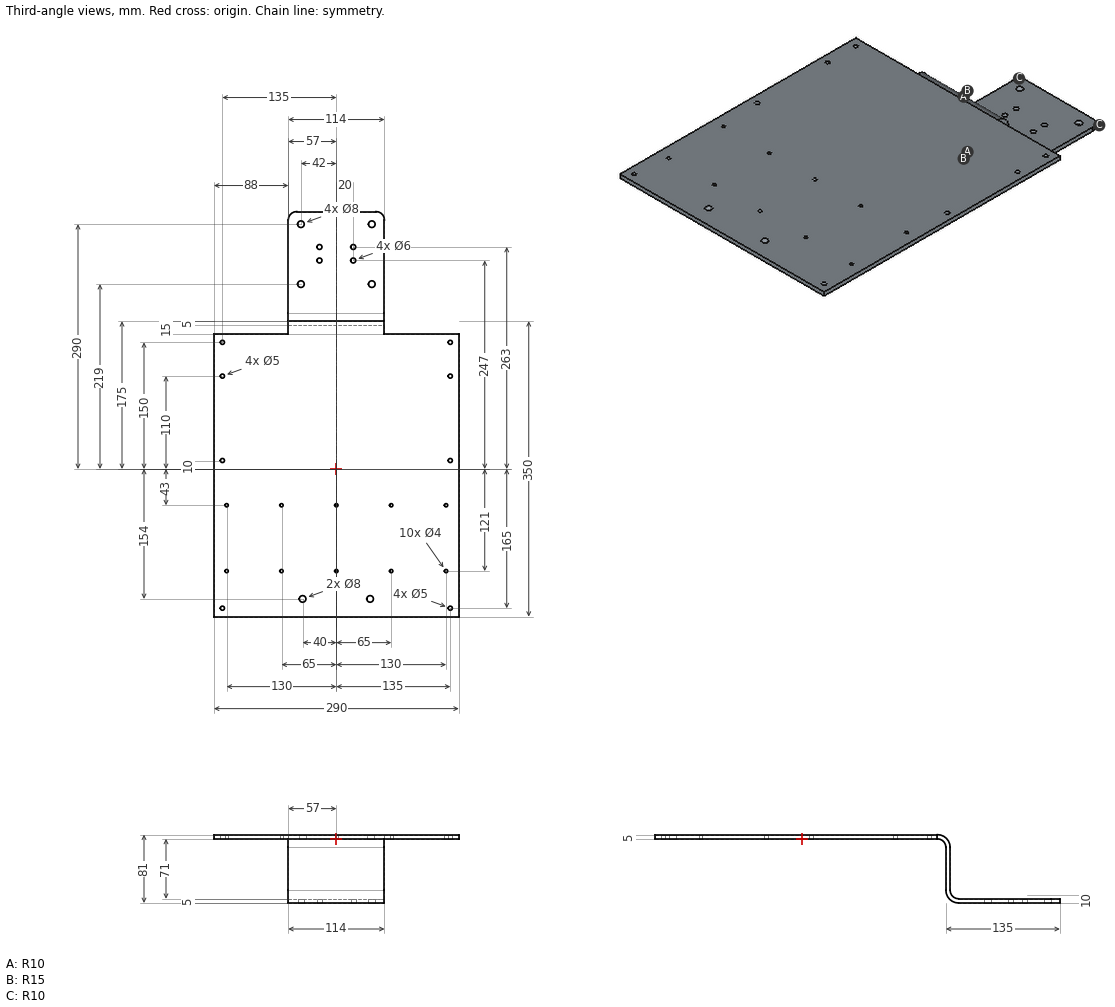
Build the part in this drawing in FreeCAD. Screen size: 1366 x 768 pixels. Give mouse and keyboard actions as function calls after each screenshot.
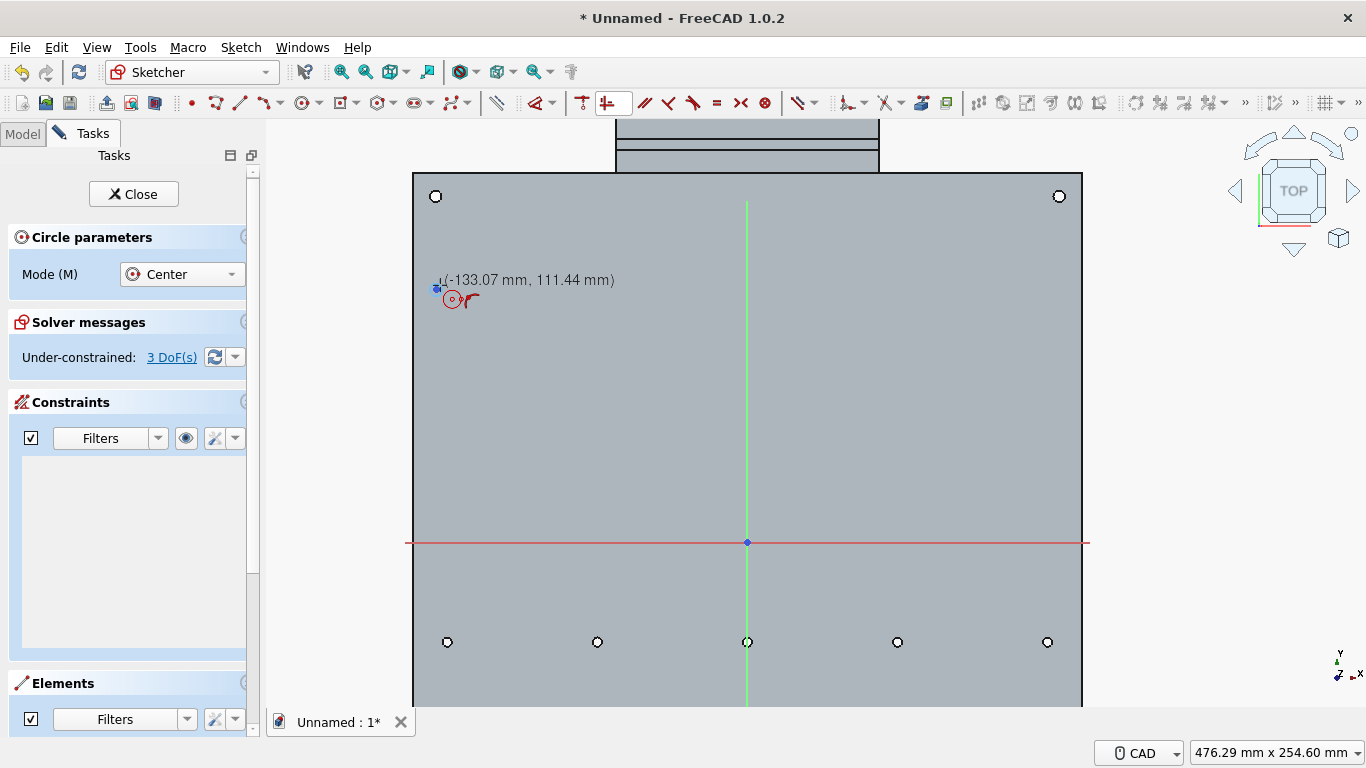
scroll(436, 520, up, 7)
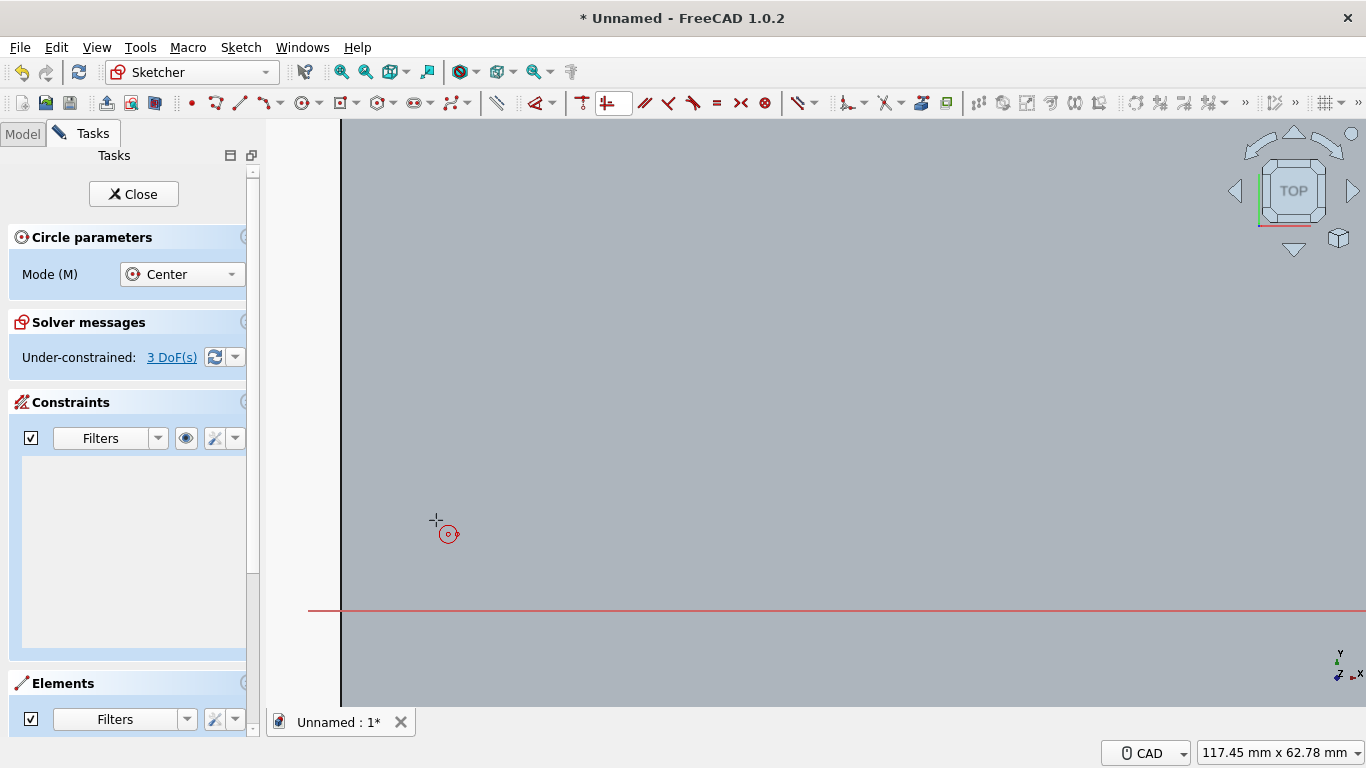
scroll(436, 521, down, 7)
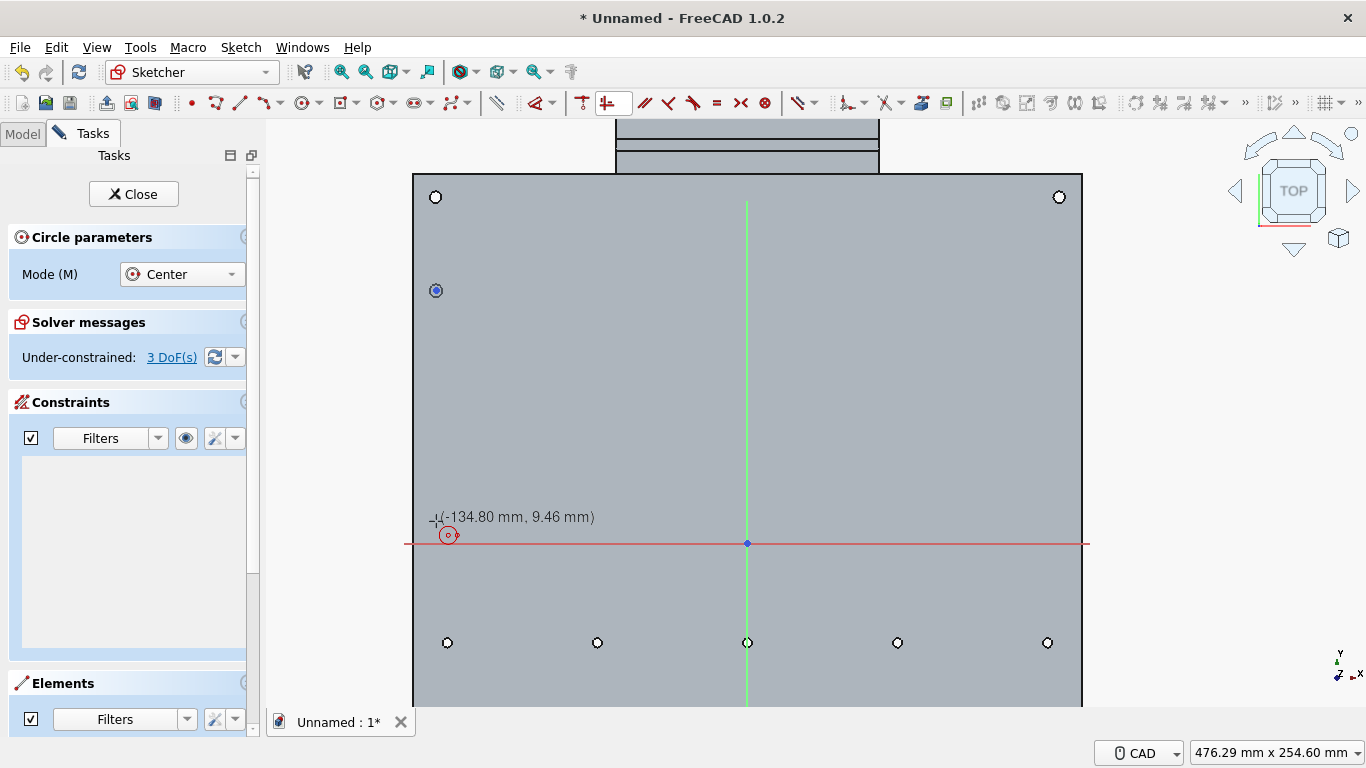
click(436, 521)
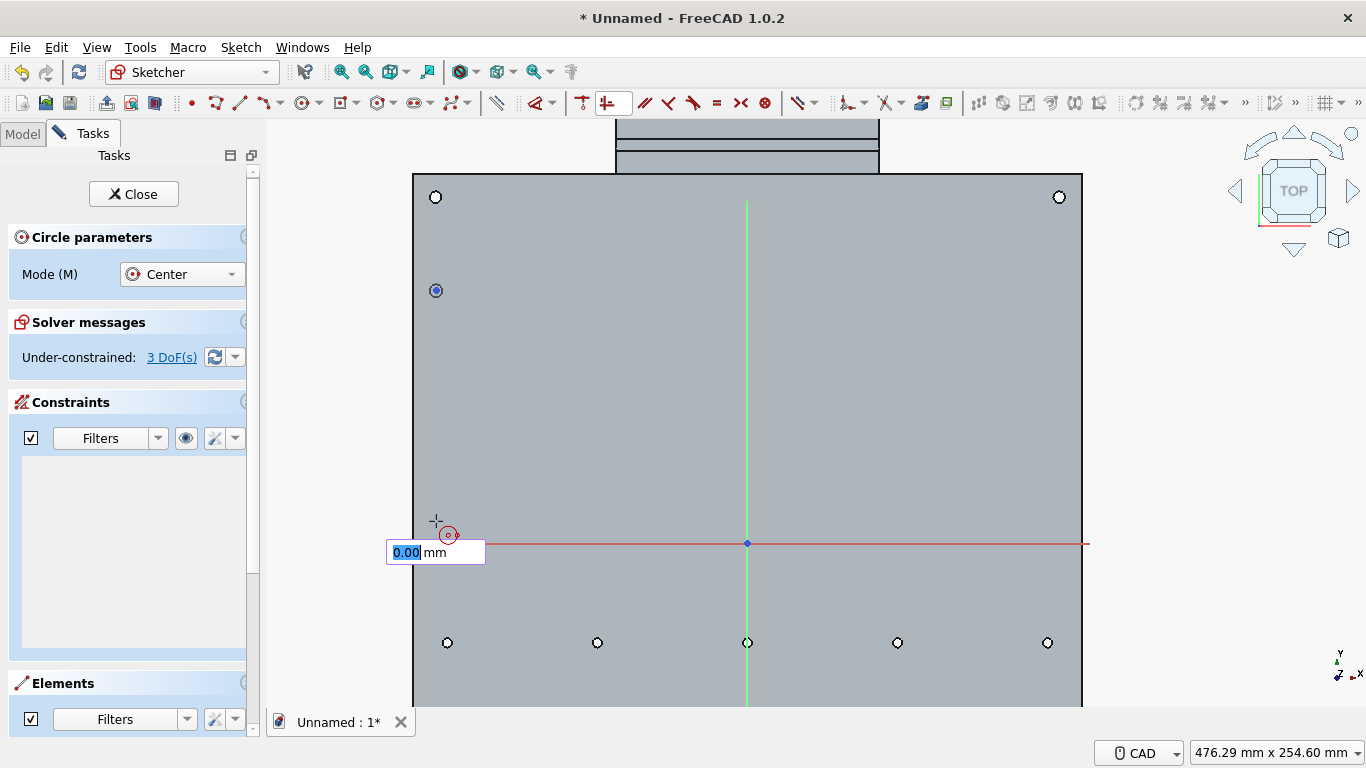
scroll(440, 516, up, 6)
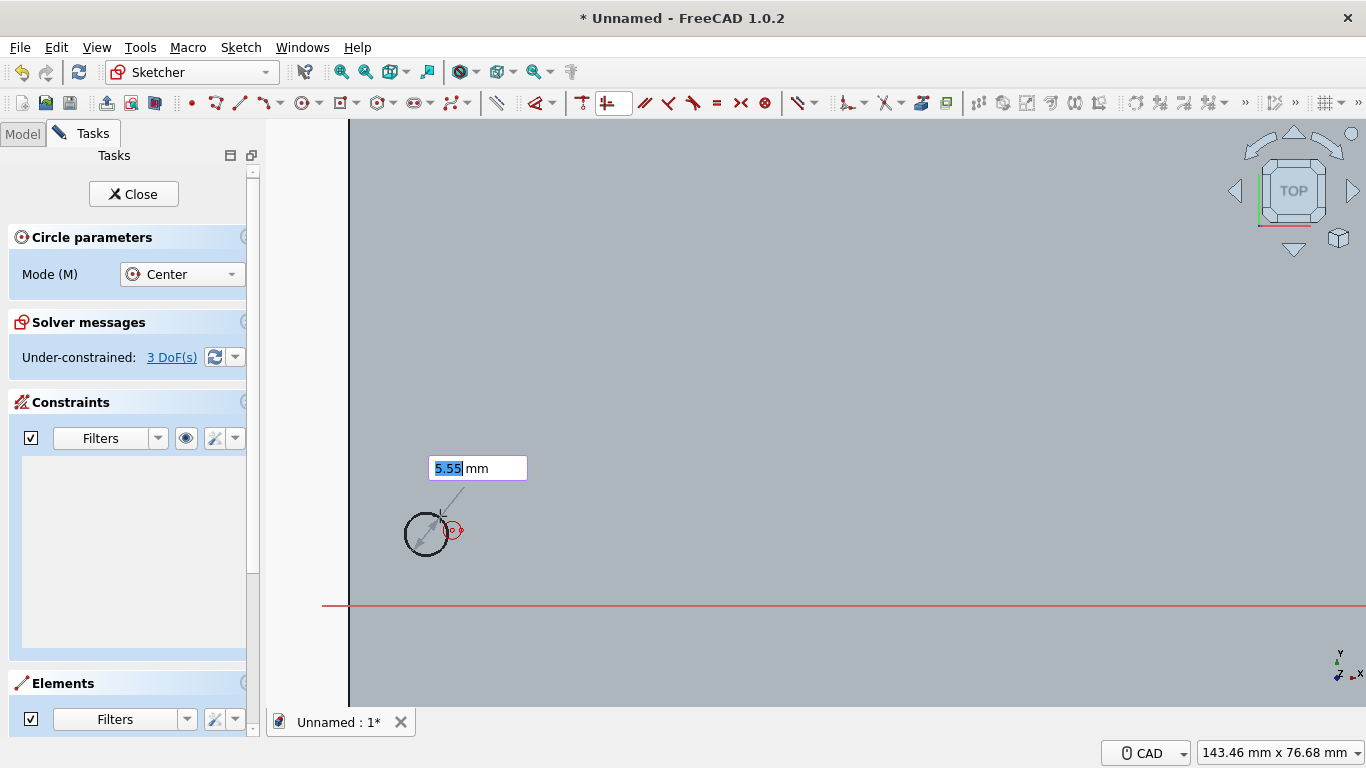
click(439, 516)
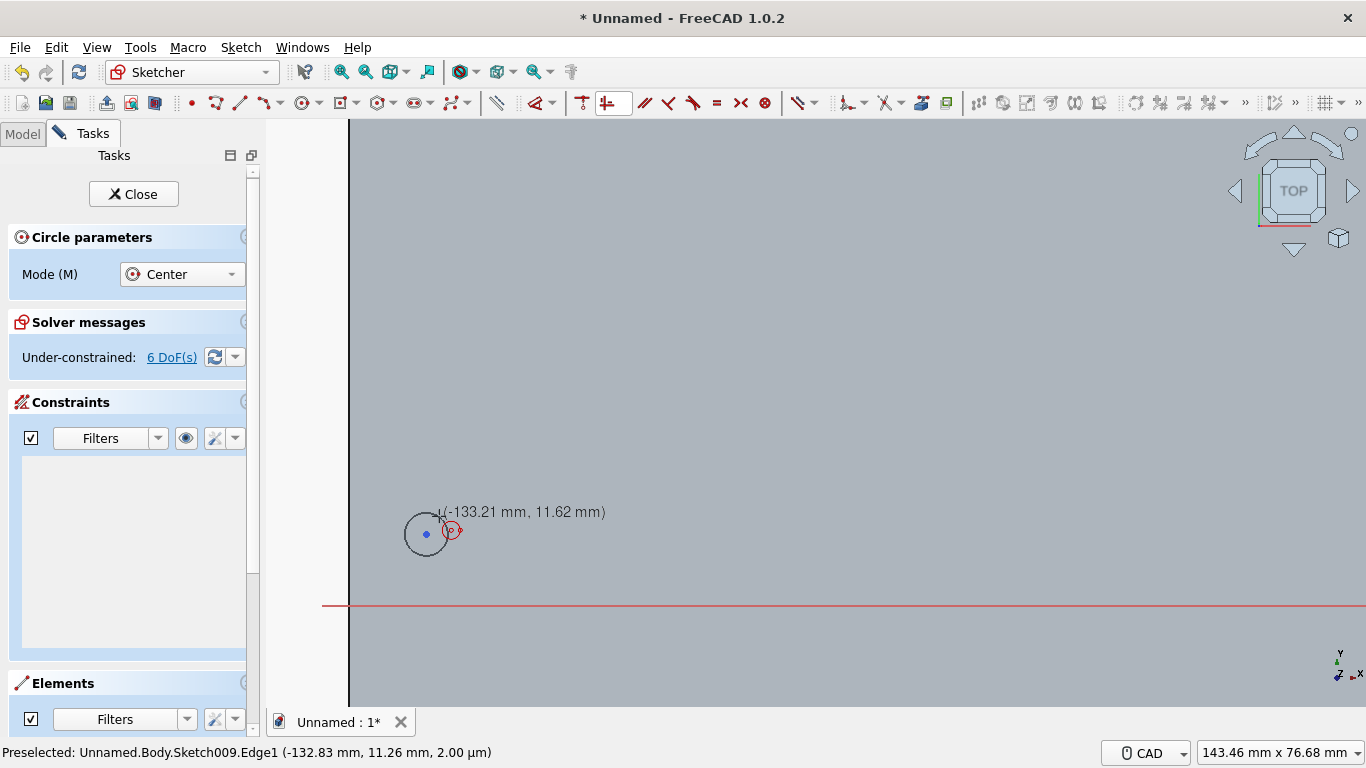
scroll(440, 516, down, 6)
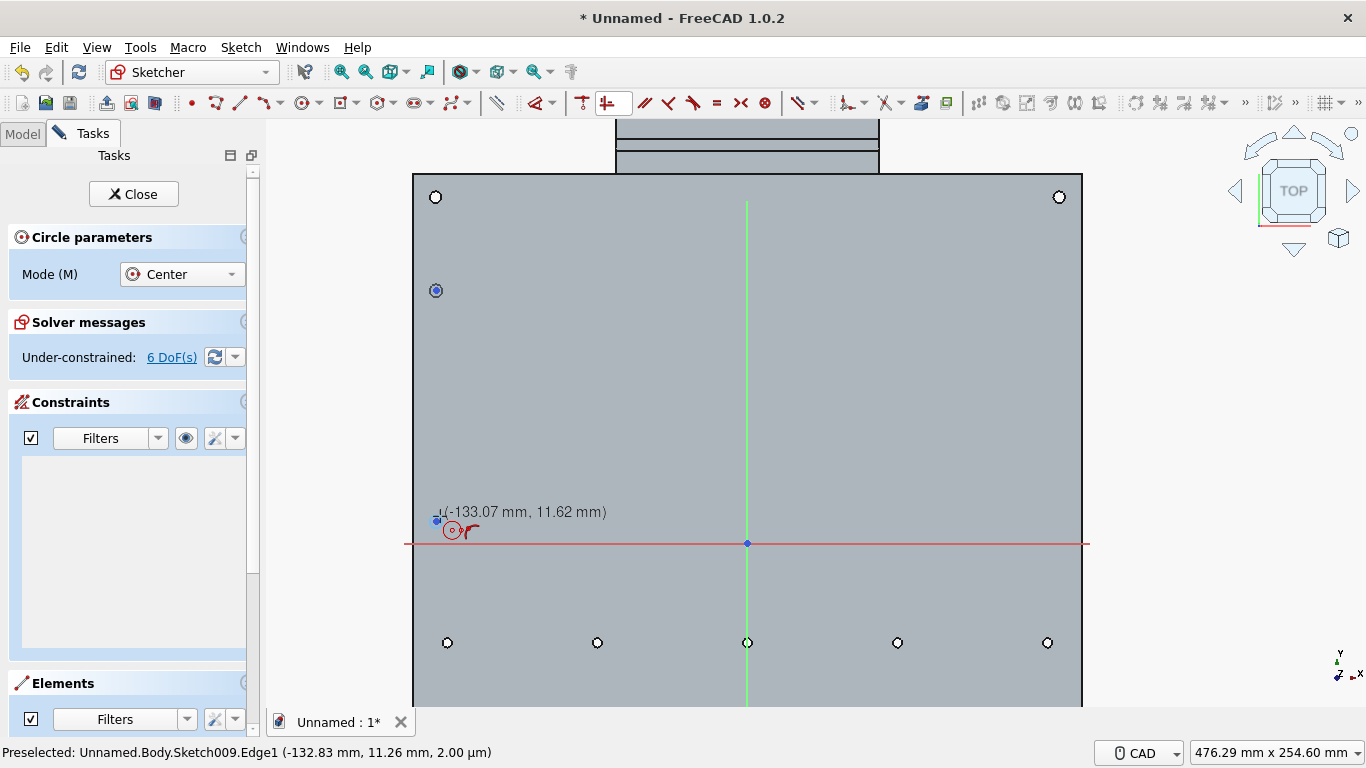
scroll(1059, 290, up, 7)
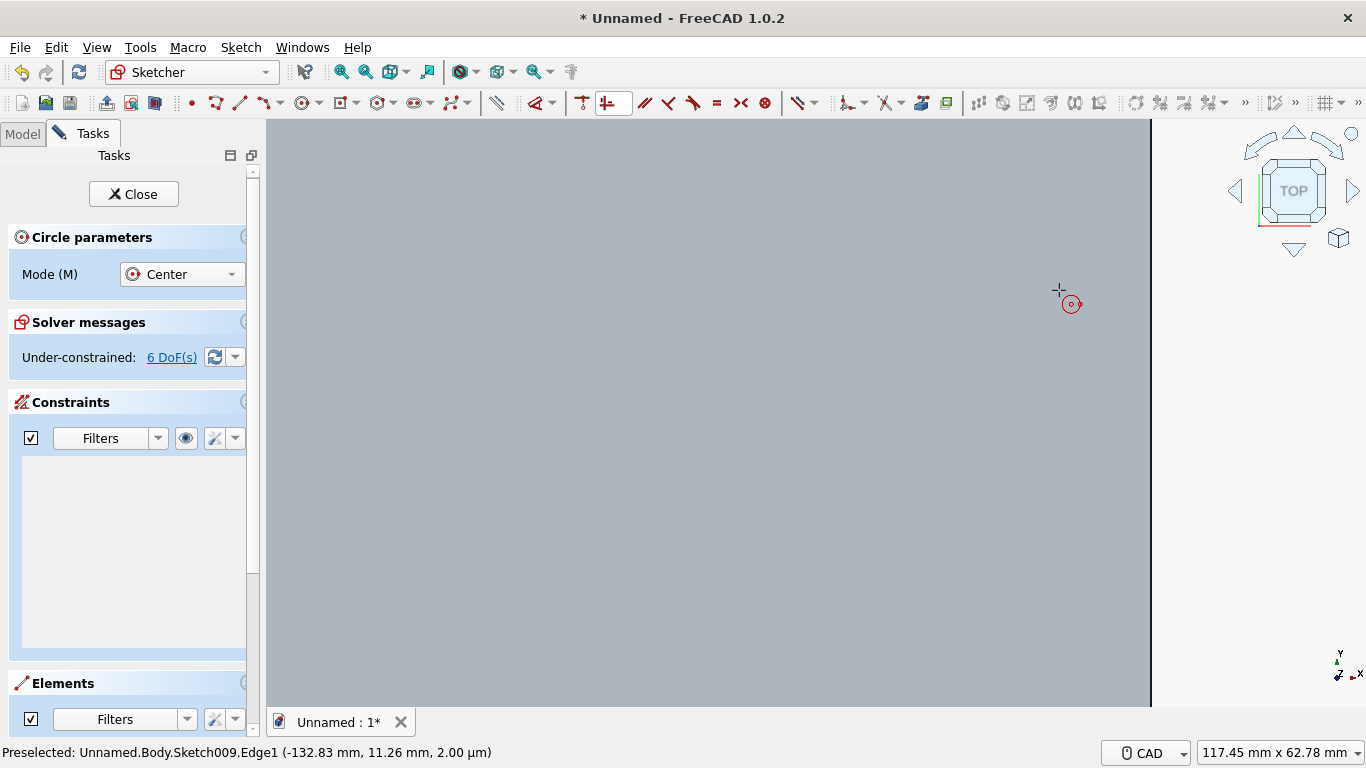
scroll(1060, 289, down, 7)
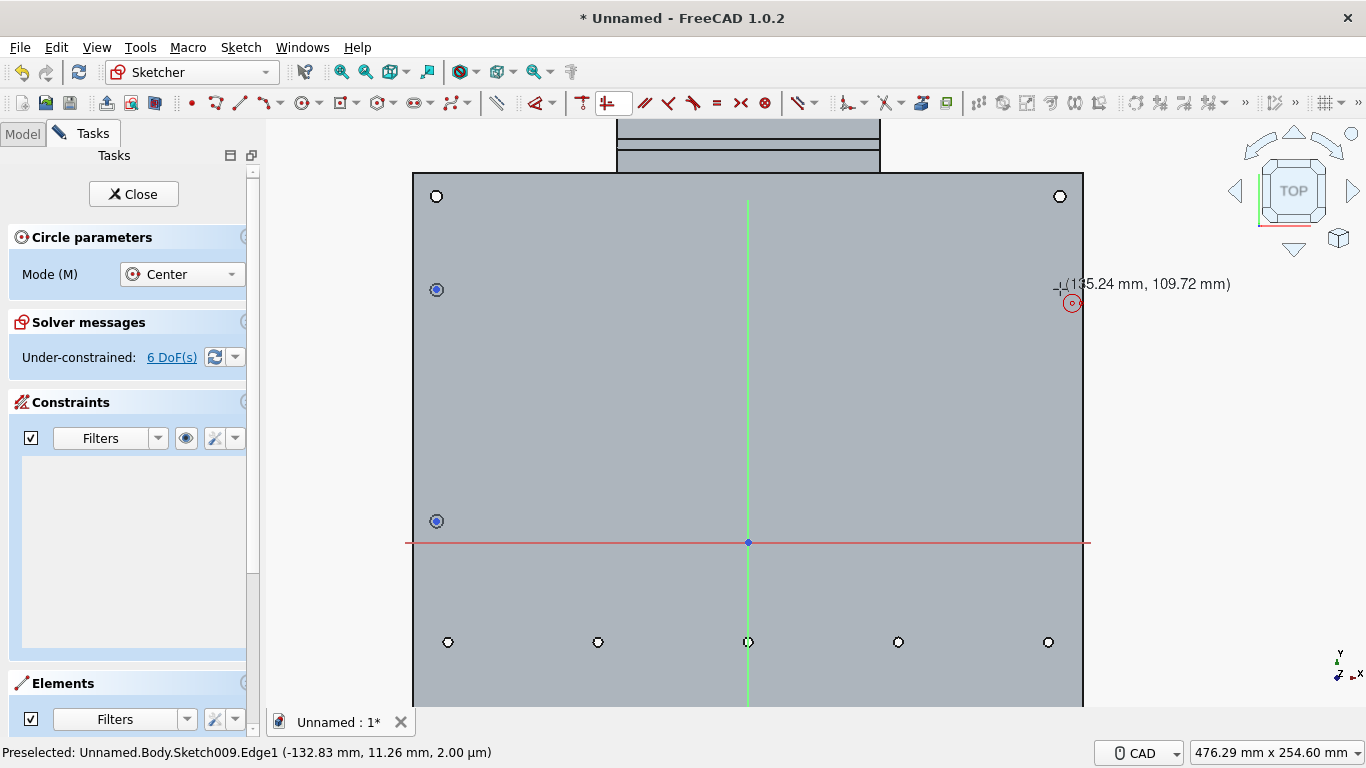
click(1060, 289)